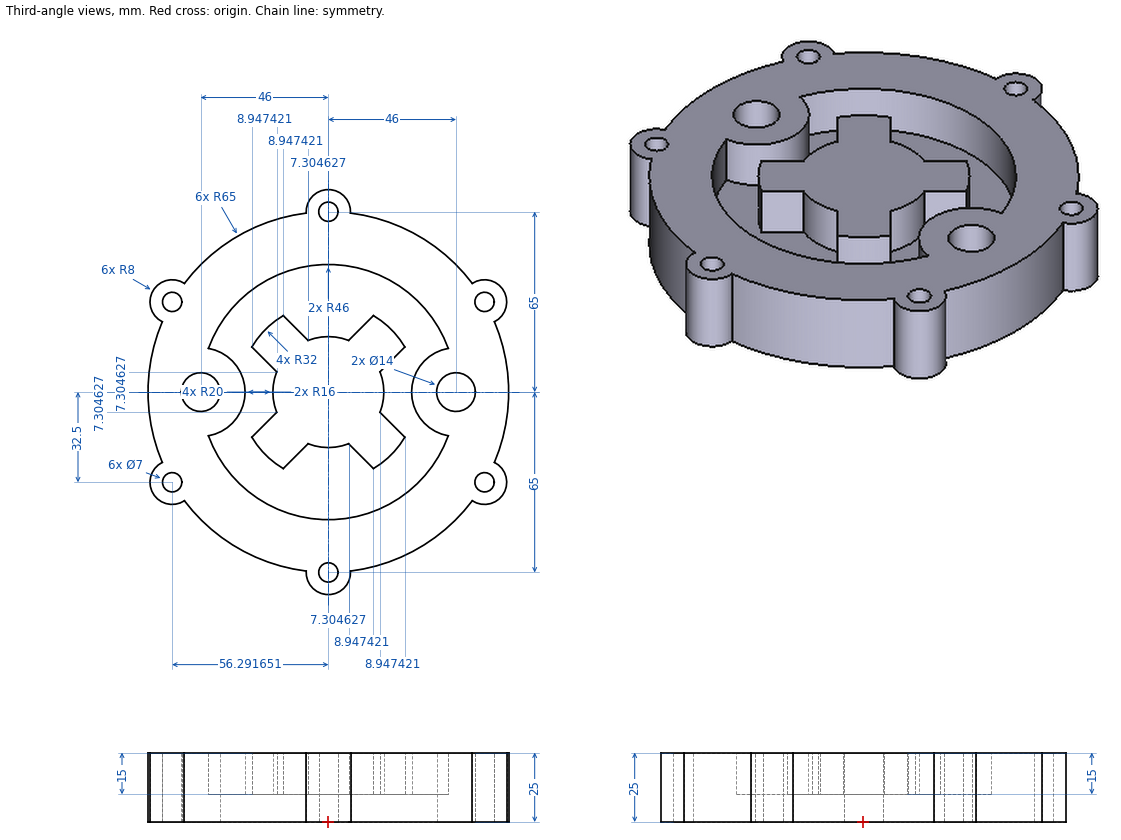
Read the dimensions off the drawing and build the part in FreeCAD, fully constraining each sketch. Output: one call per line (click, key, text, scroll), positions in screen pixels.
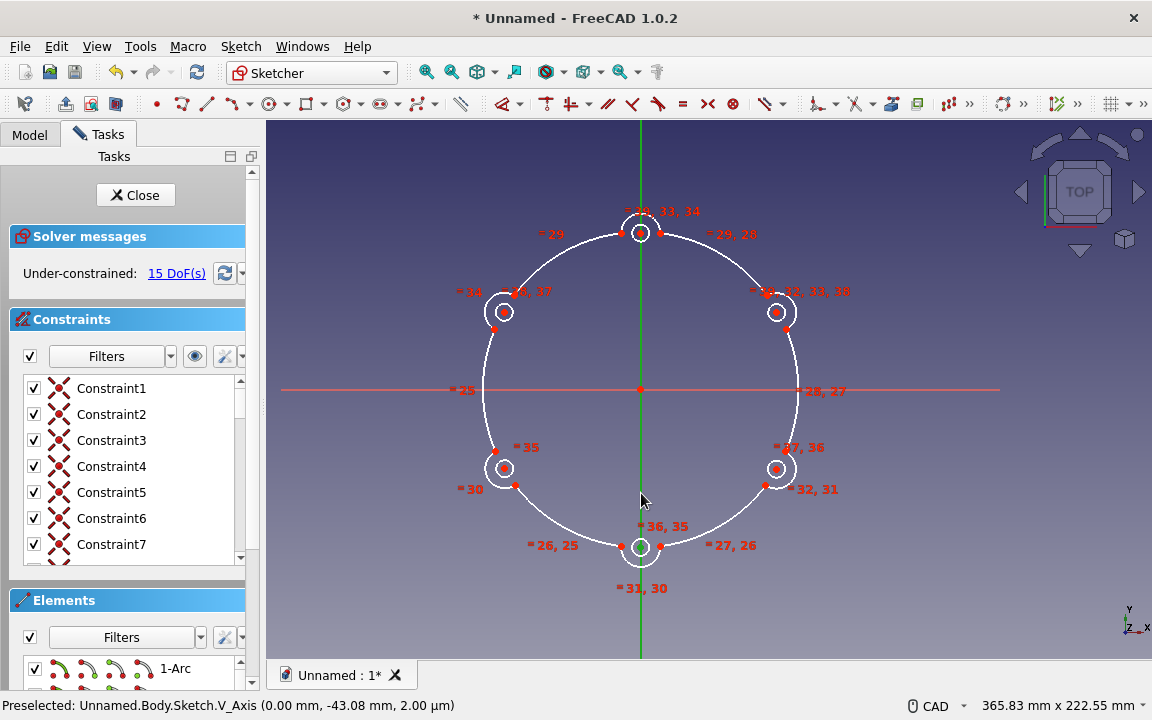
click(546, 104)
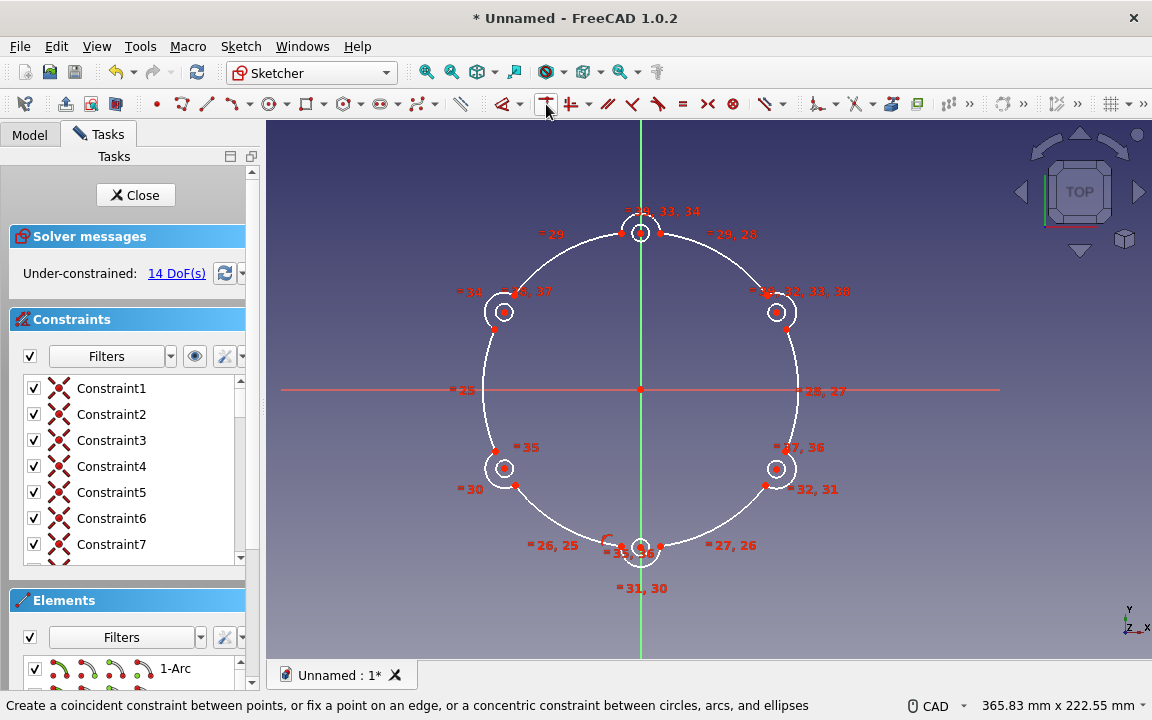
click(641, 233)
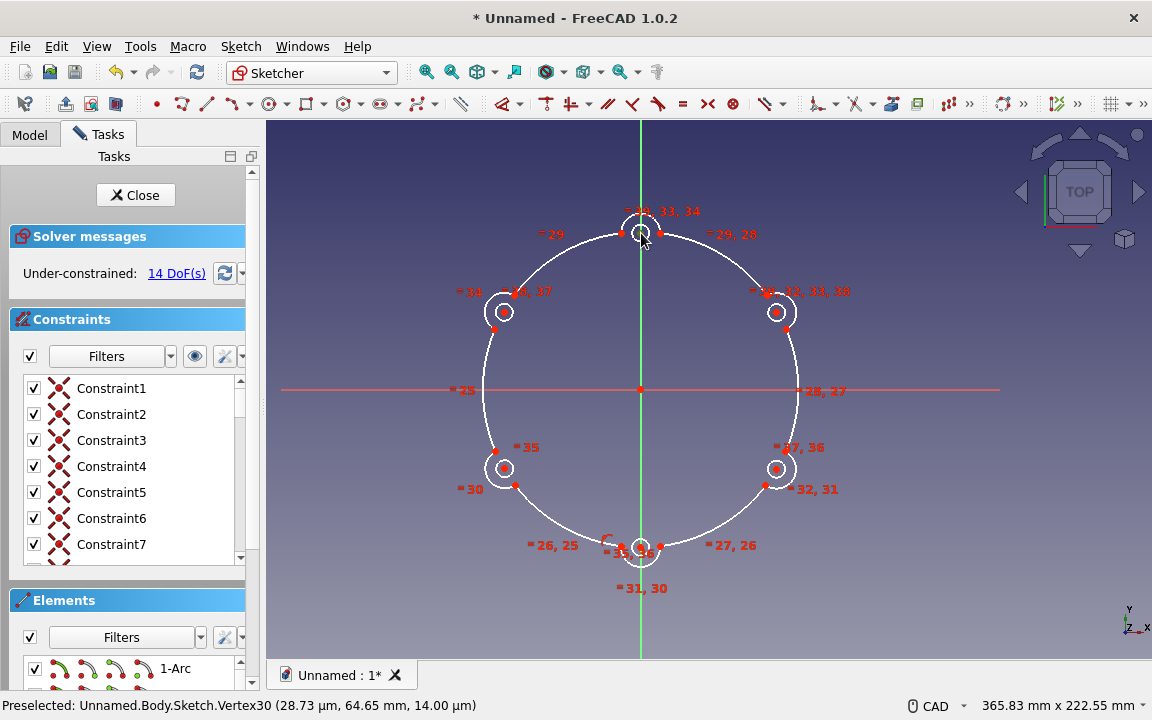
click(641, 493)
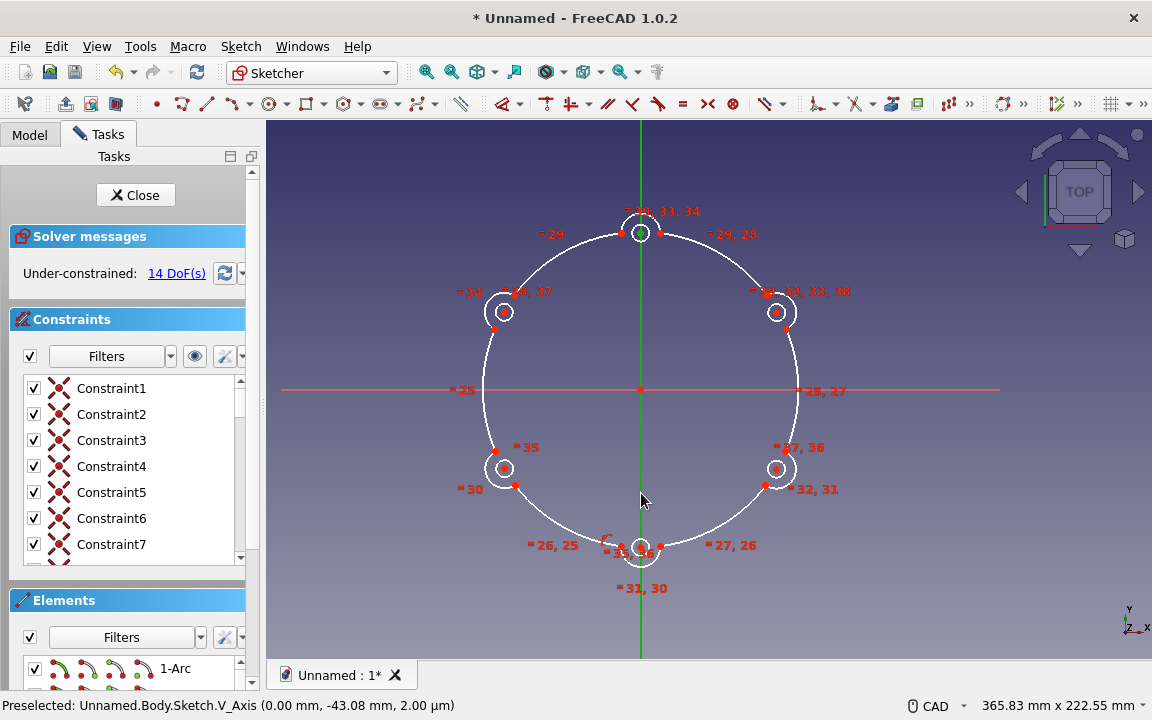
click(546, 104)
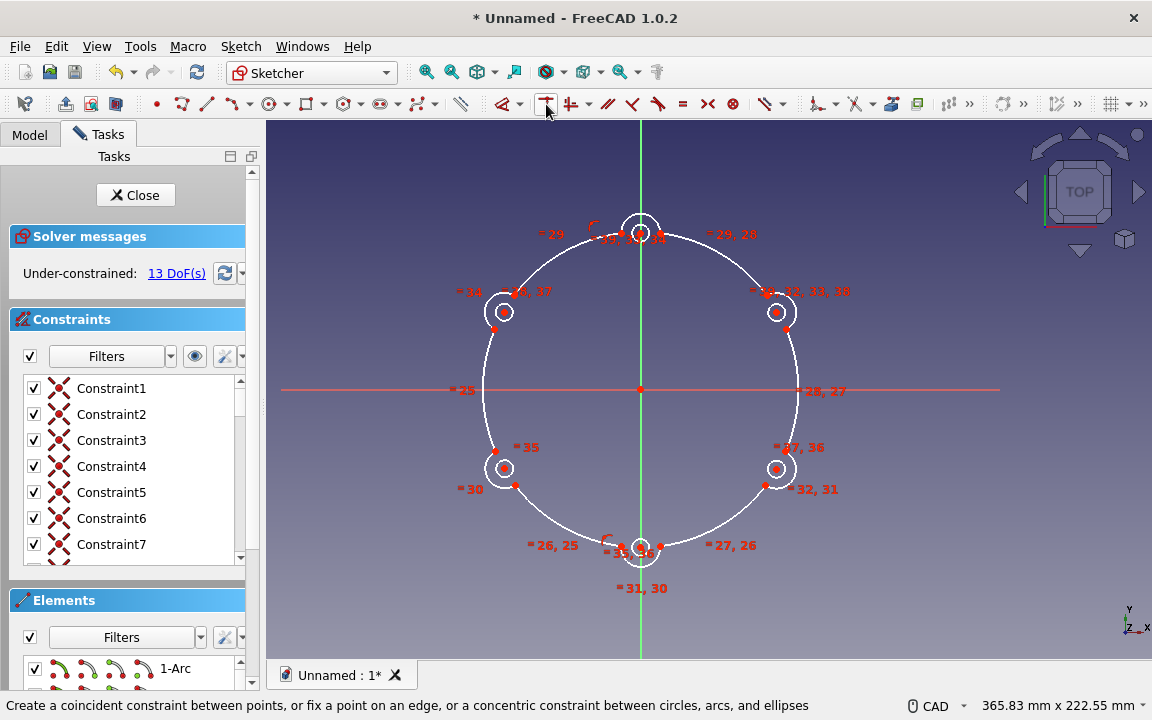
click(505, 469)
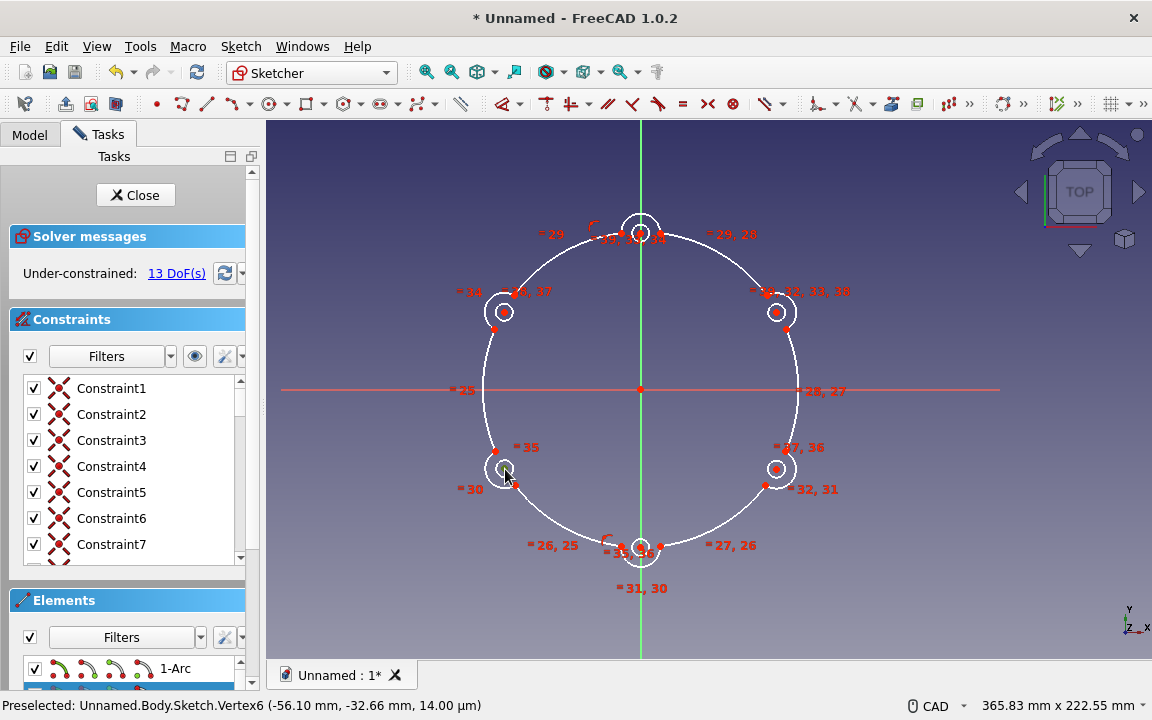
click(777, 469)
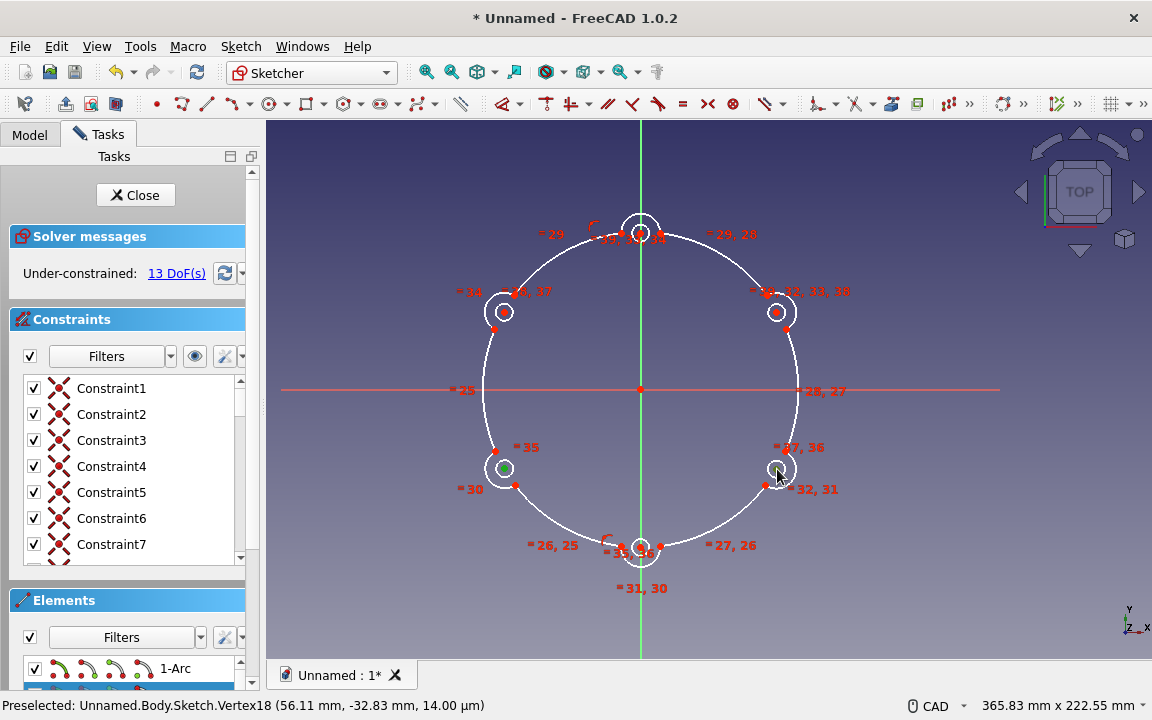
click(641, 493)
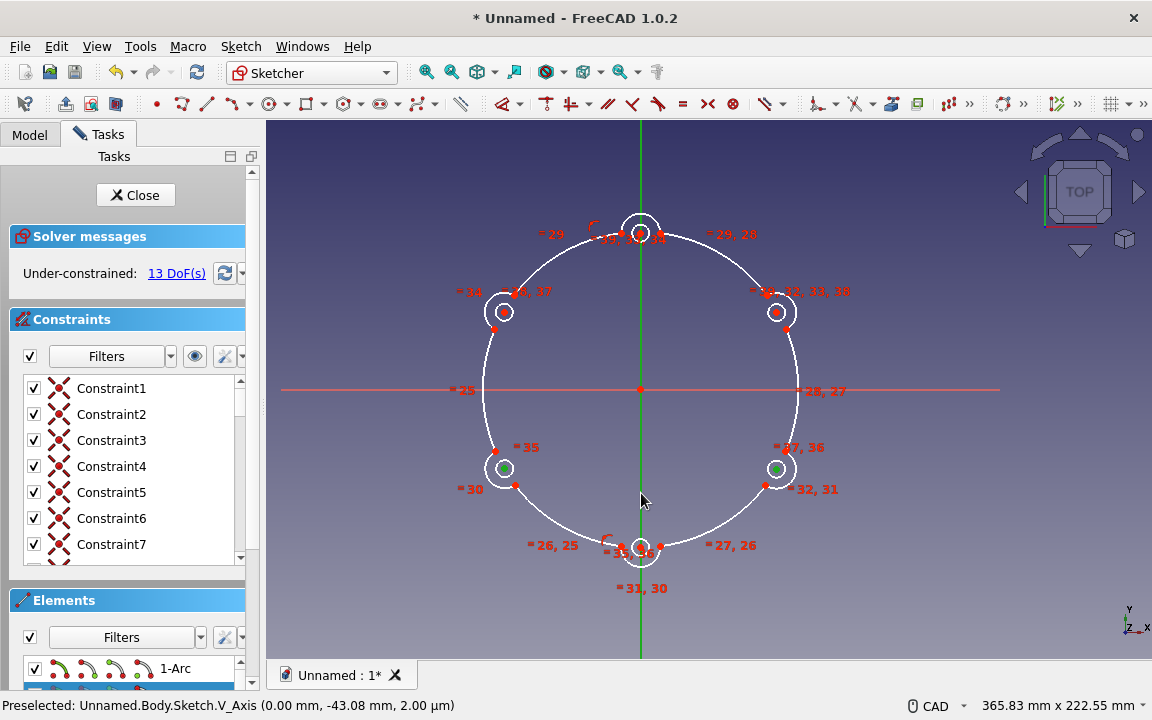
click(708, 104)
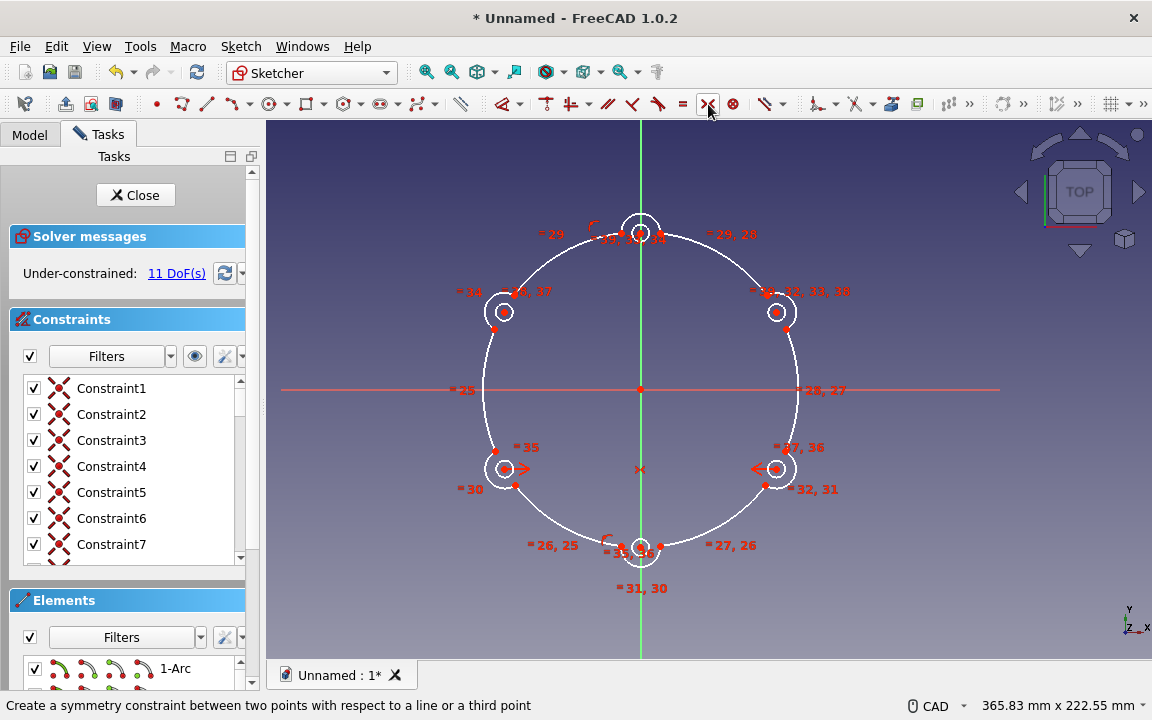
click(777, 469)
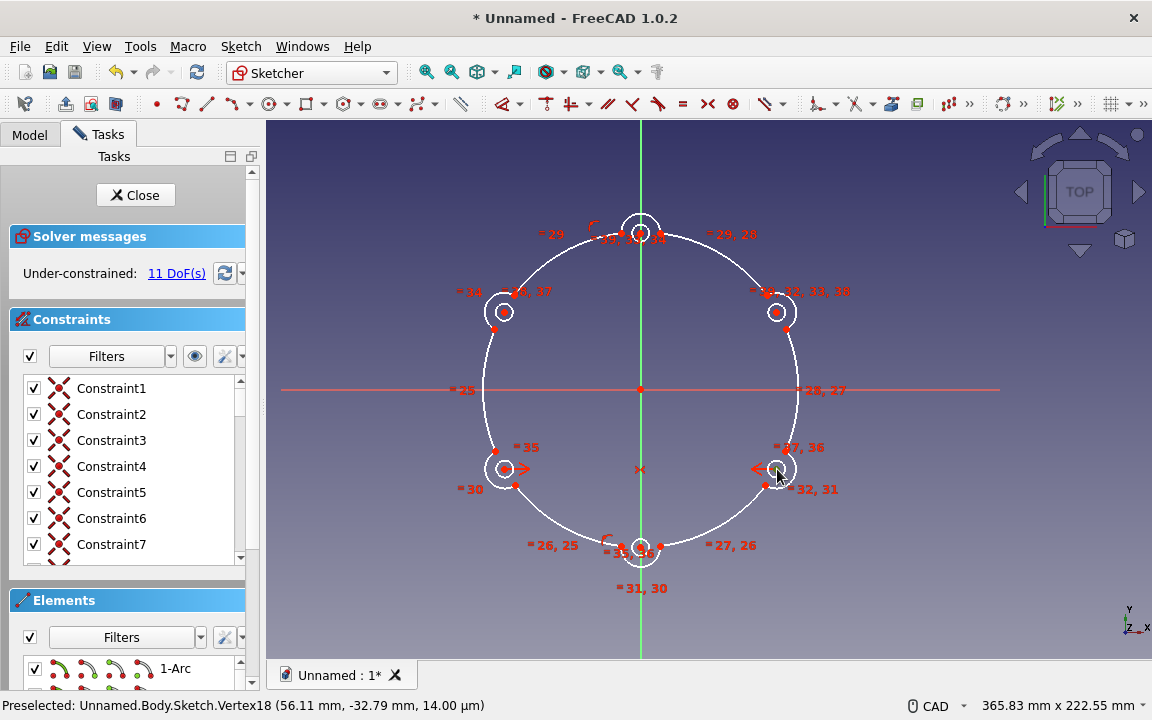
click(777, 313)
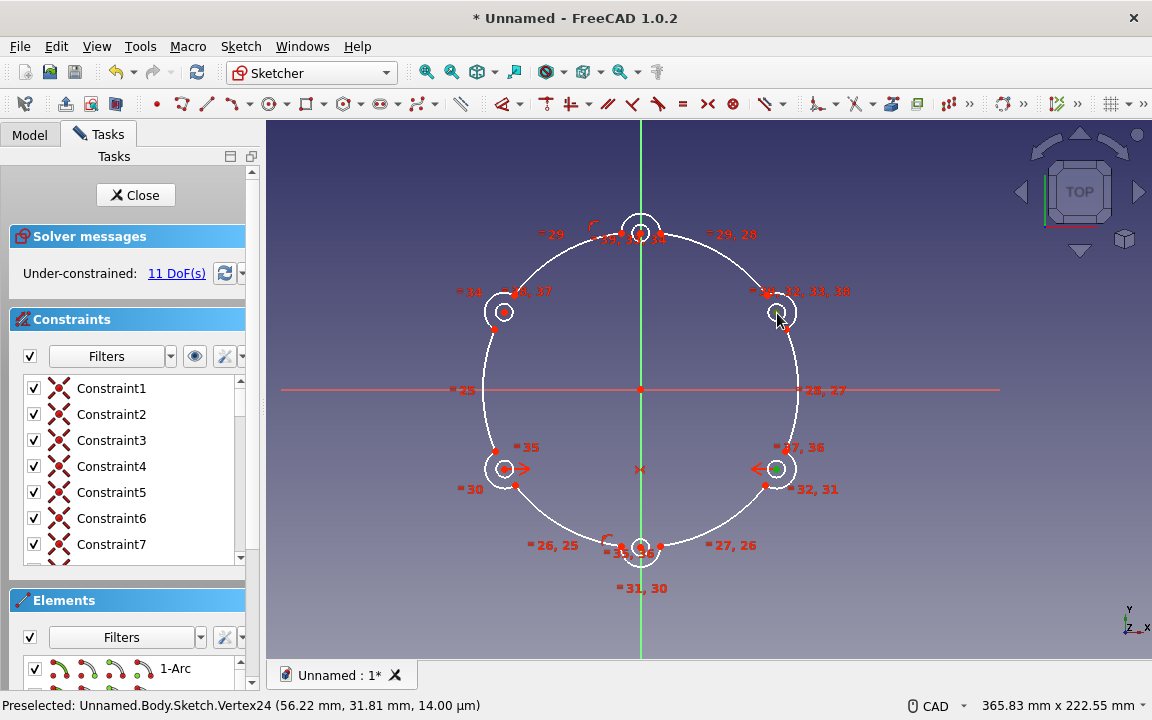
click(344, 390)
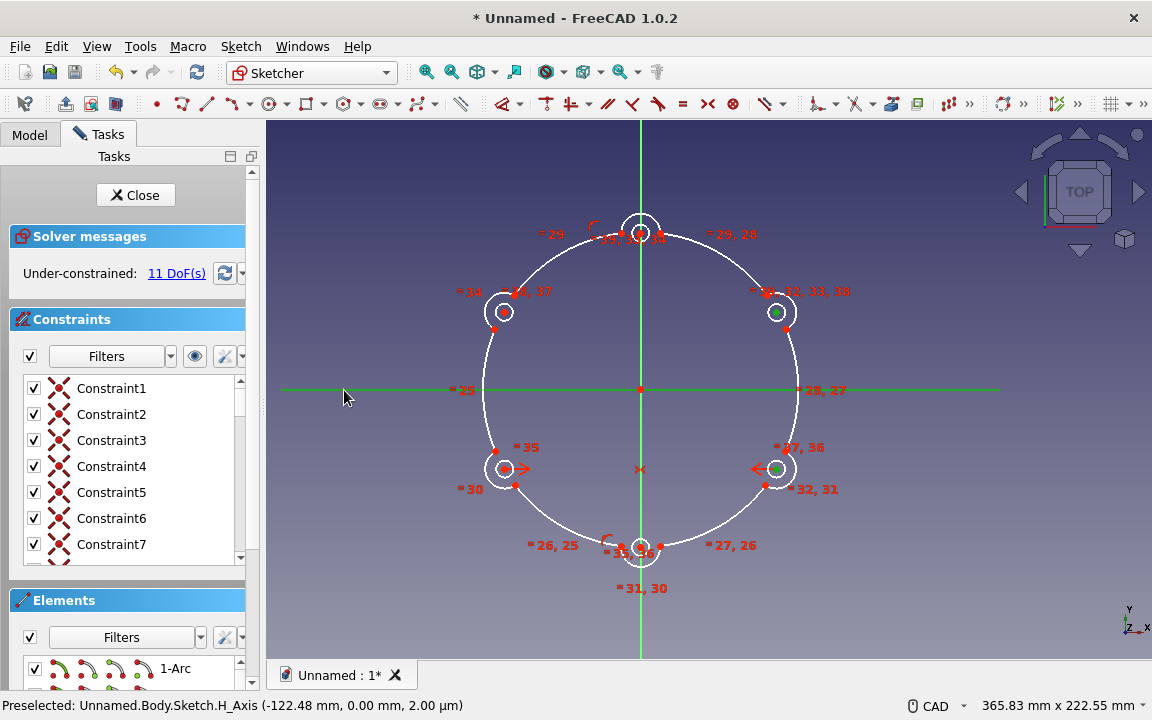
click(708, 104)